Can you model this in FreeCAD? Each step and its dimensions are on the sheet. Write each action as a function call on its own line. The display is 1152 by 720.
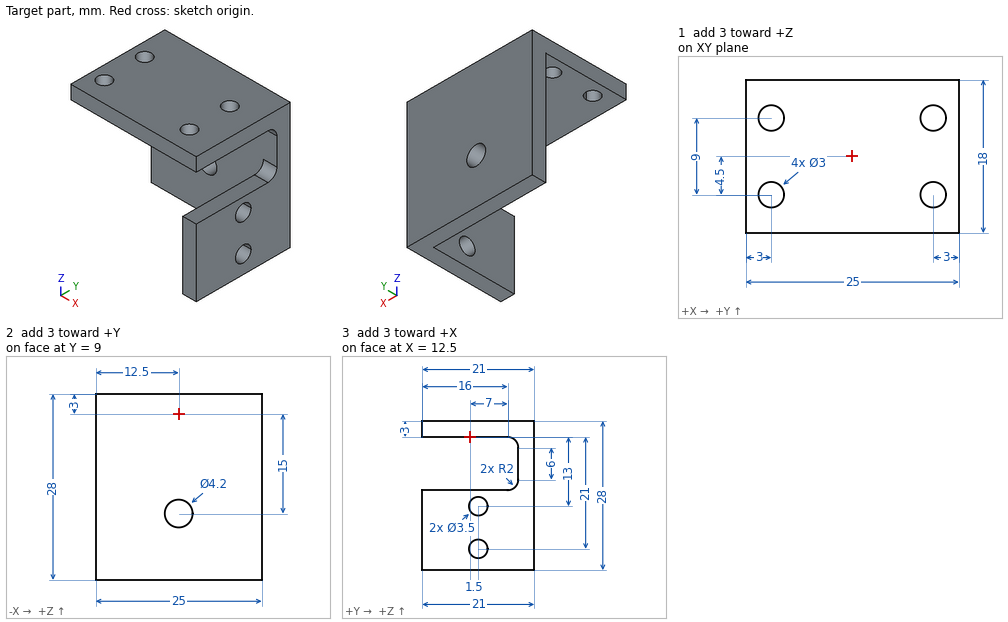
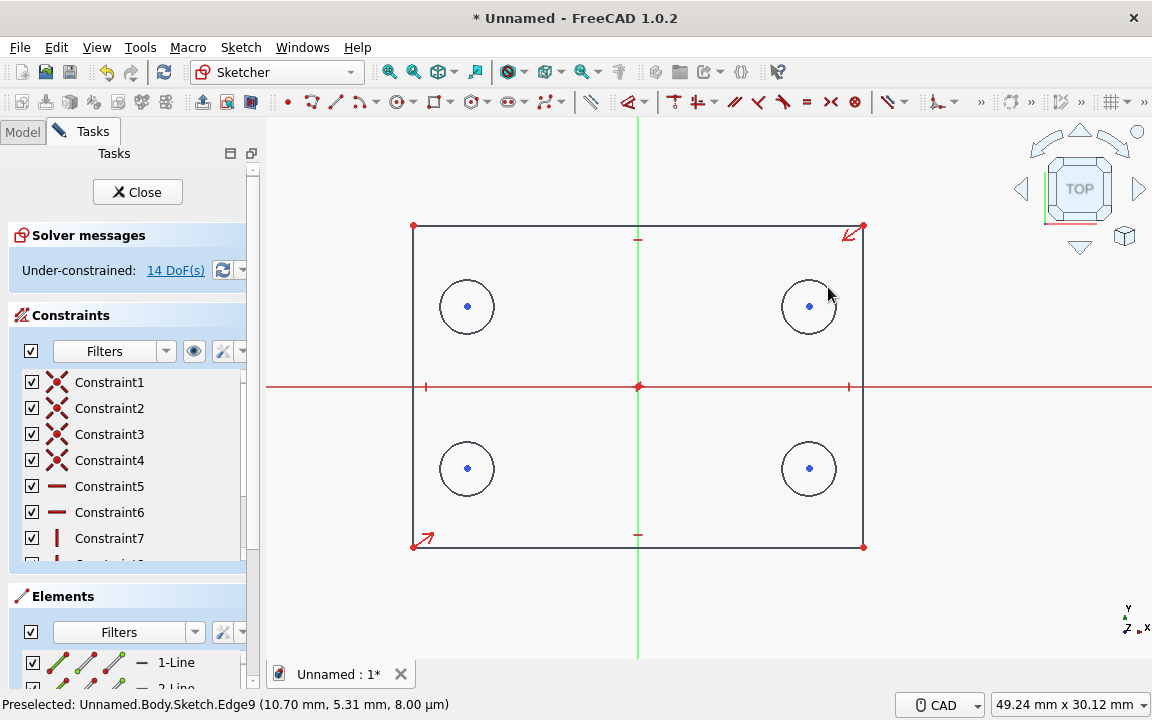
click(486, 450)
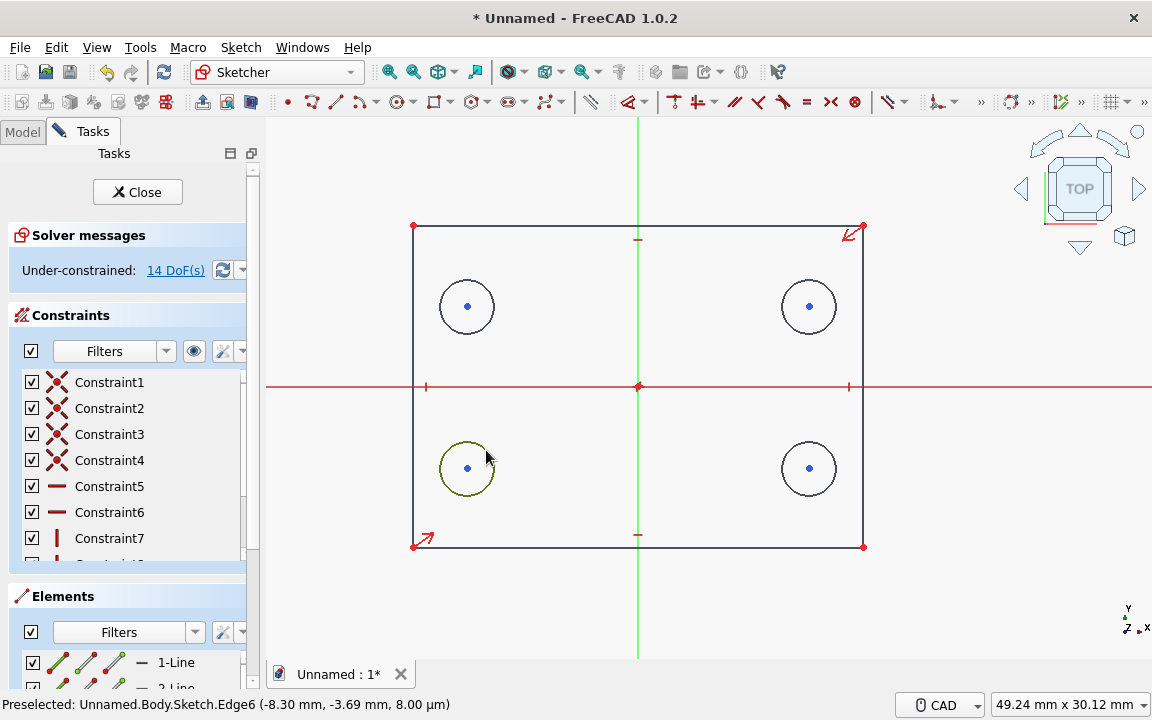
click(828, 450)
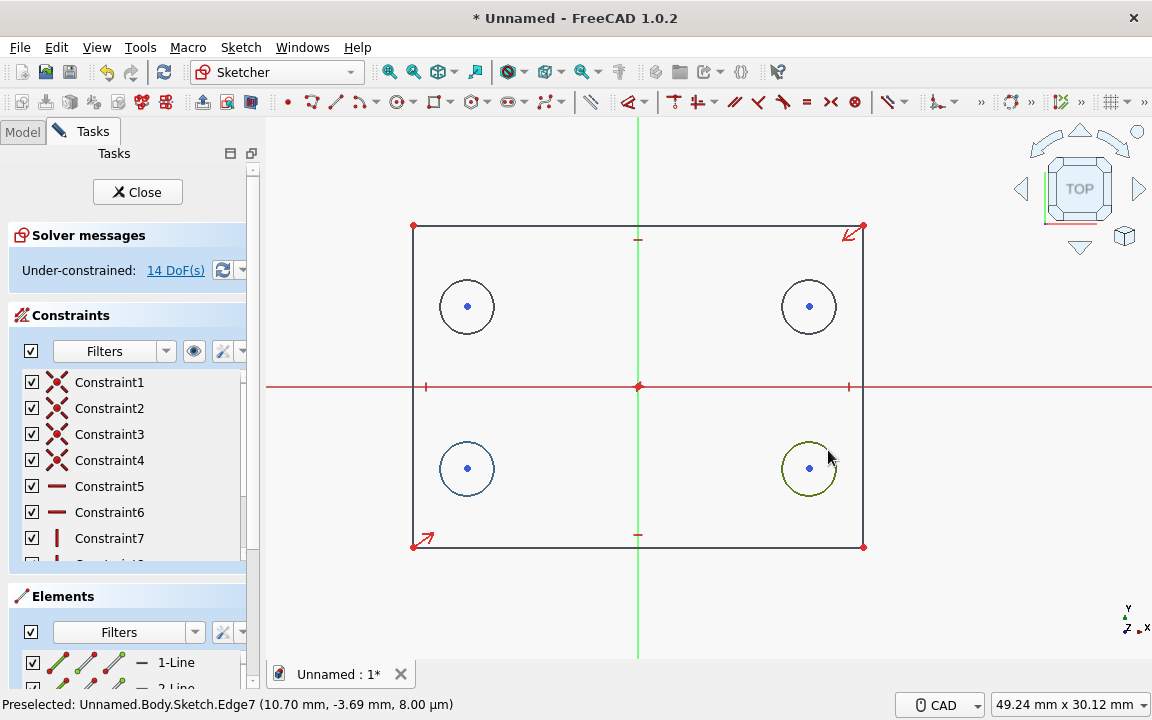
click(486, 288)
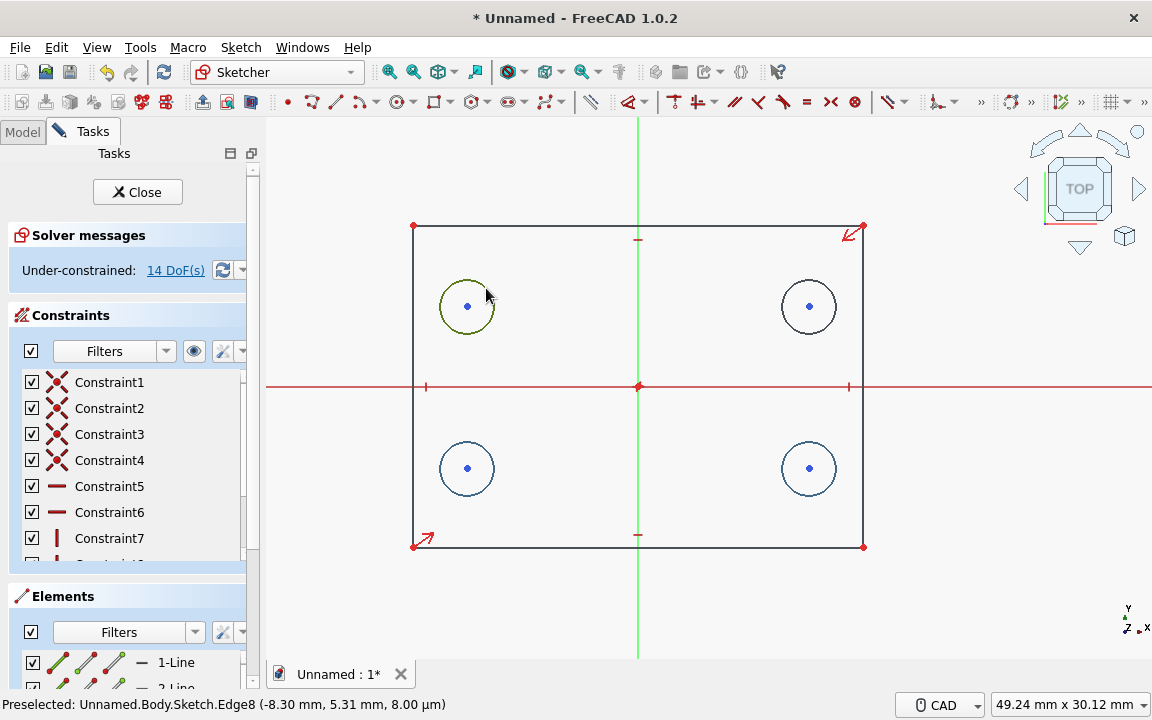
click(828, 288)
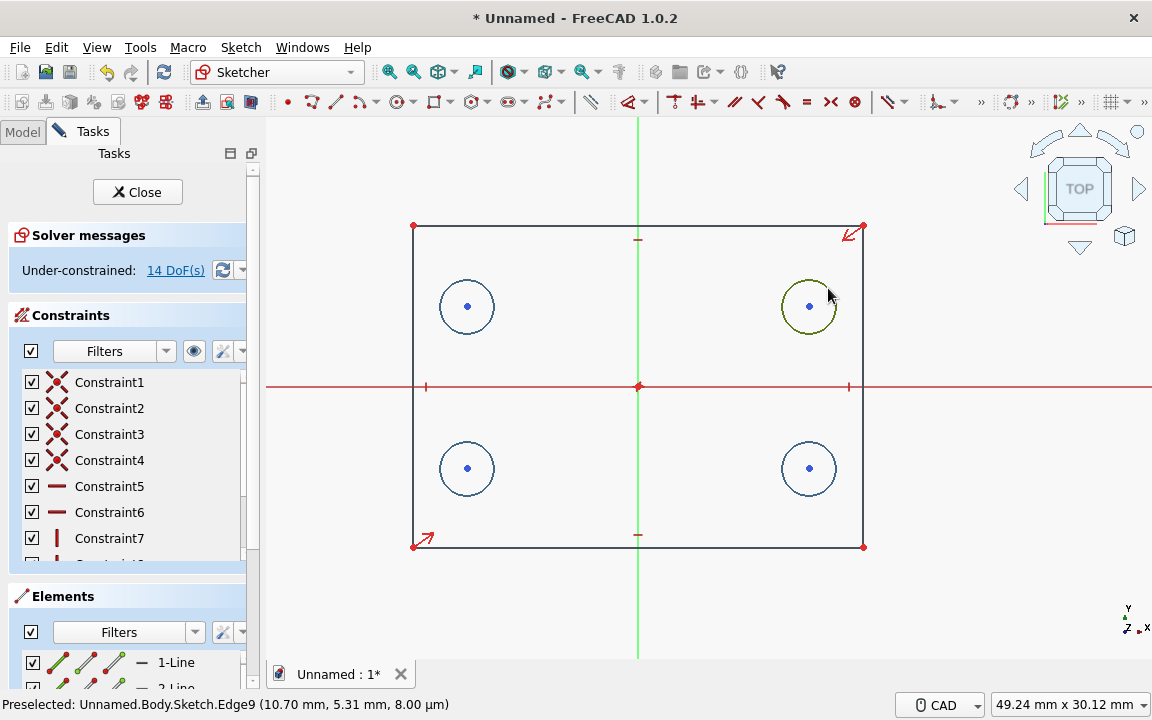
click(808, 102)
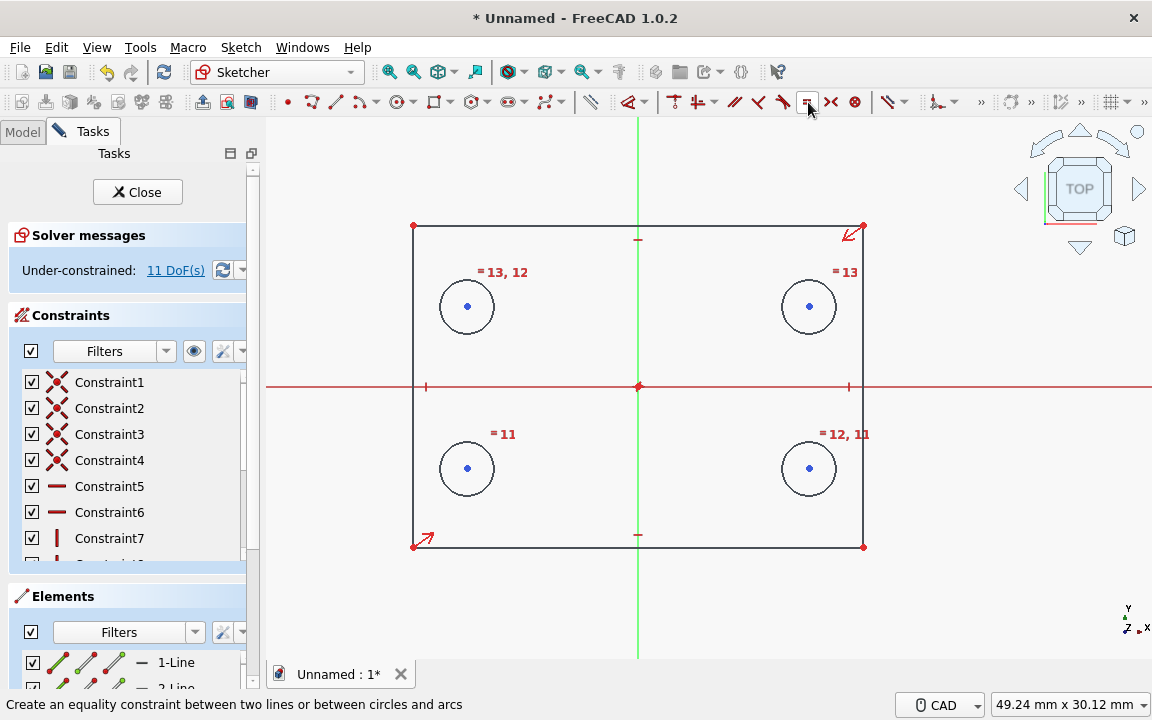
click(467, 469)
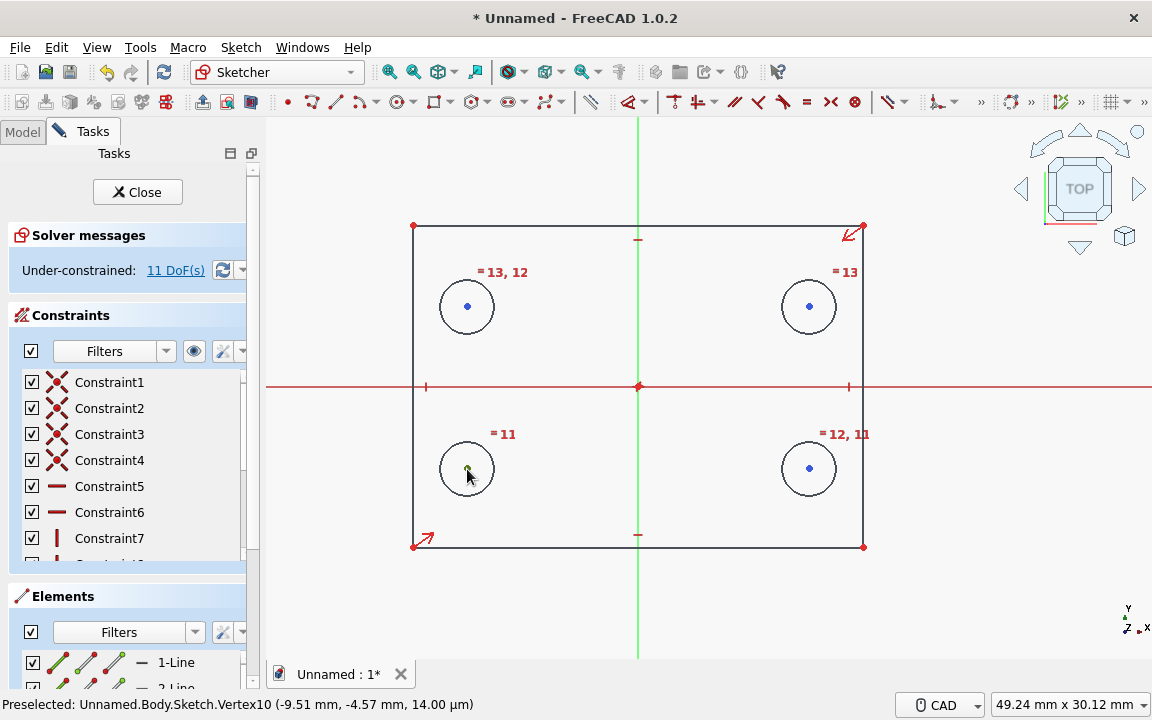
click(809, 469)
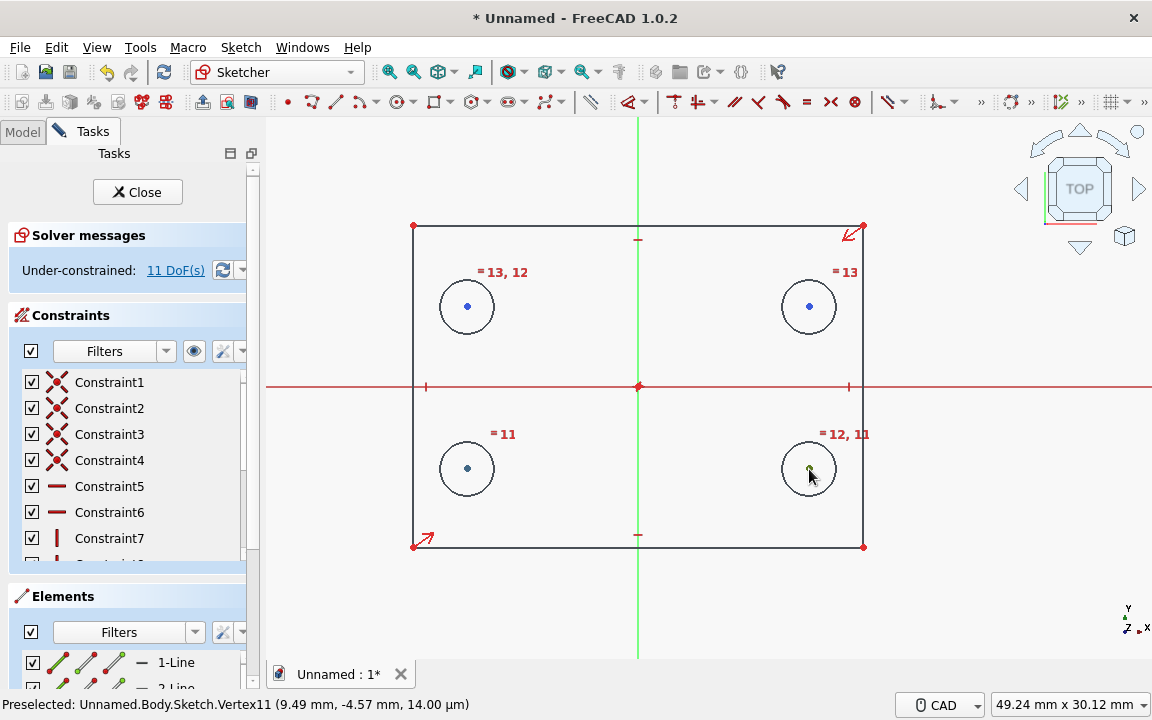
key(h)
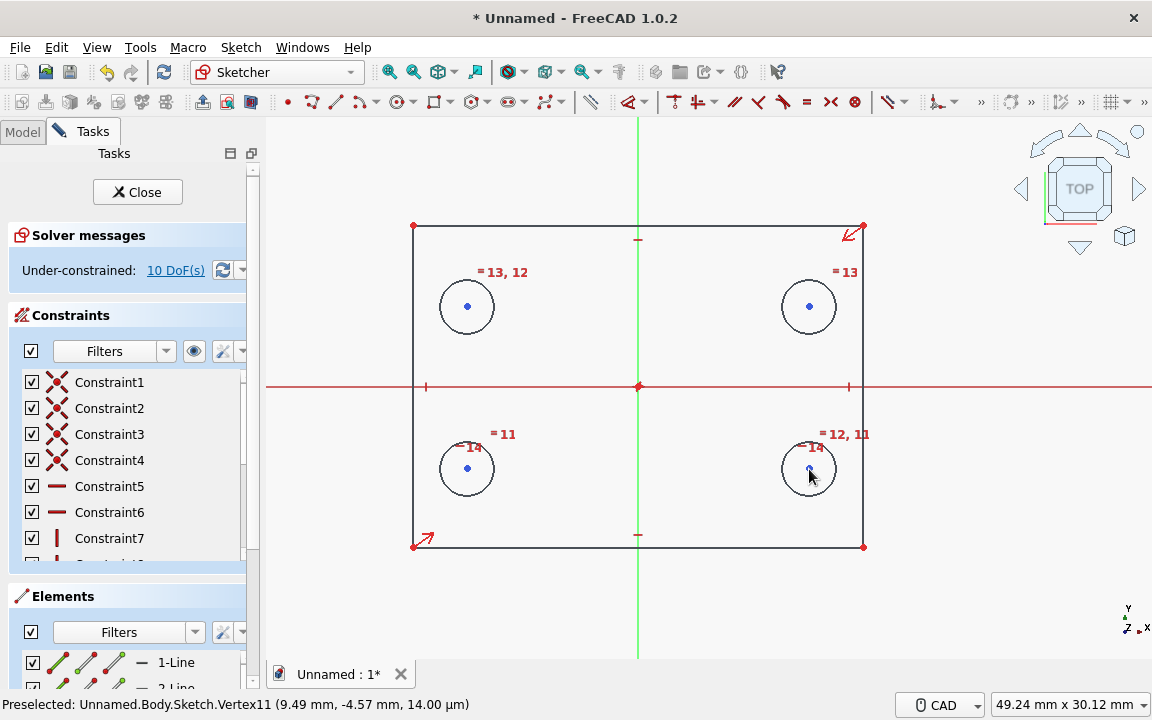
click(467, 469)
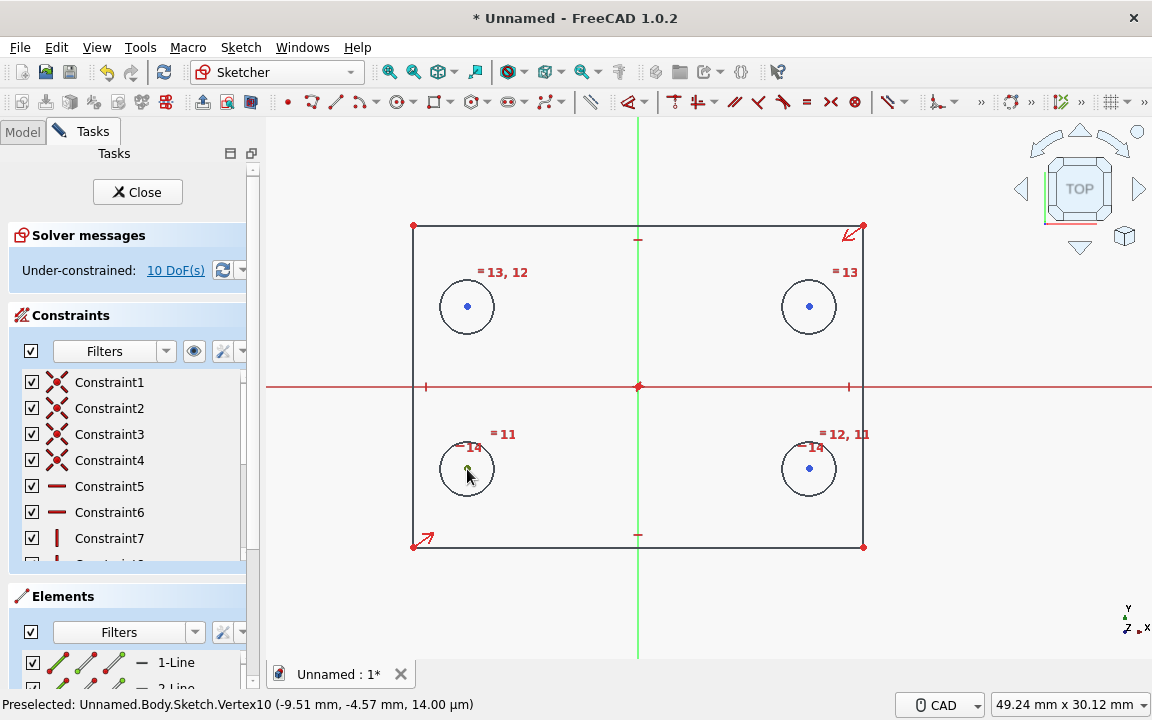
click(467, 307)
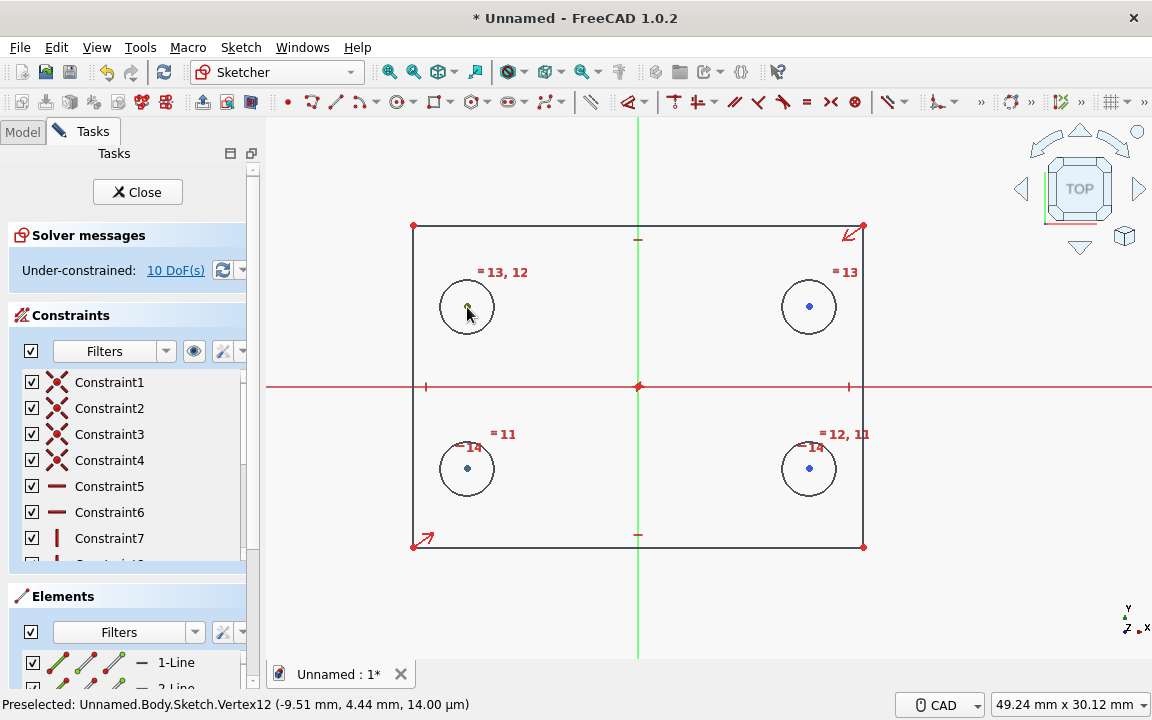
click(716, 102)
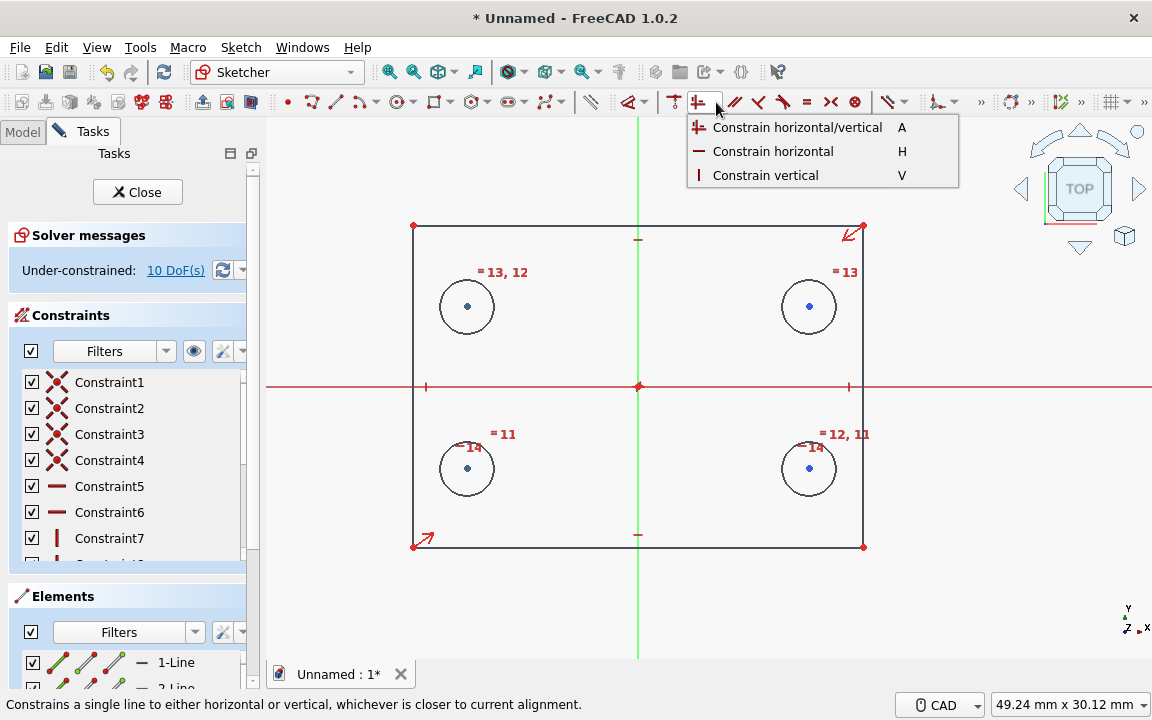
click(823, 175)